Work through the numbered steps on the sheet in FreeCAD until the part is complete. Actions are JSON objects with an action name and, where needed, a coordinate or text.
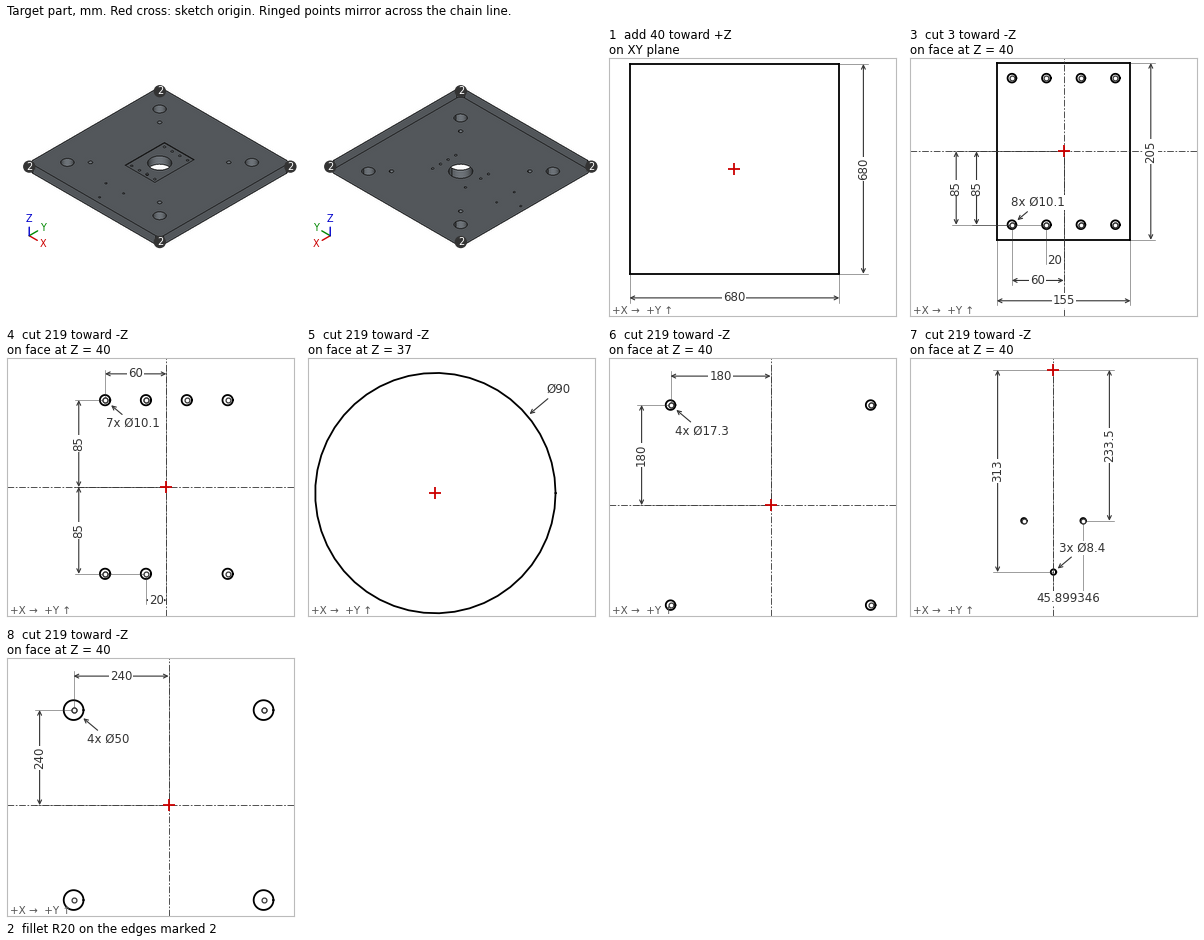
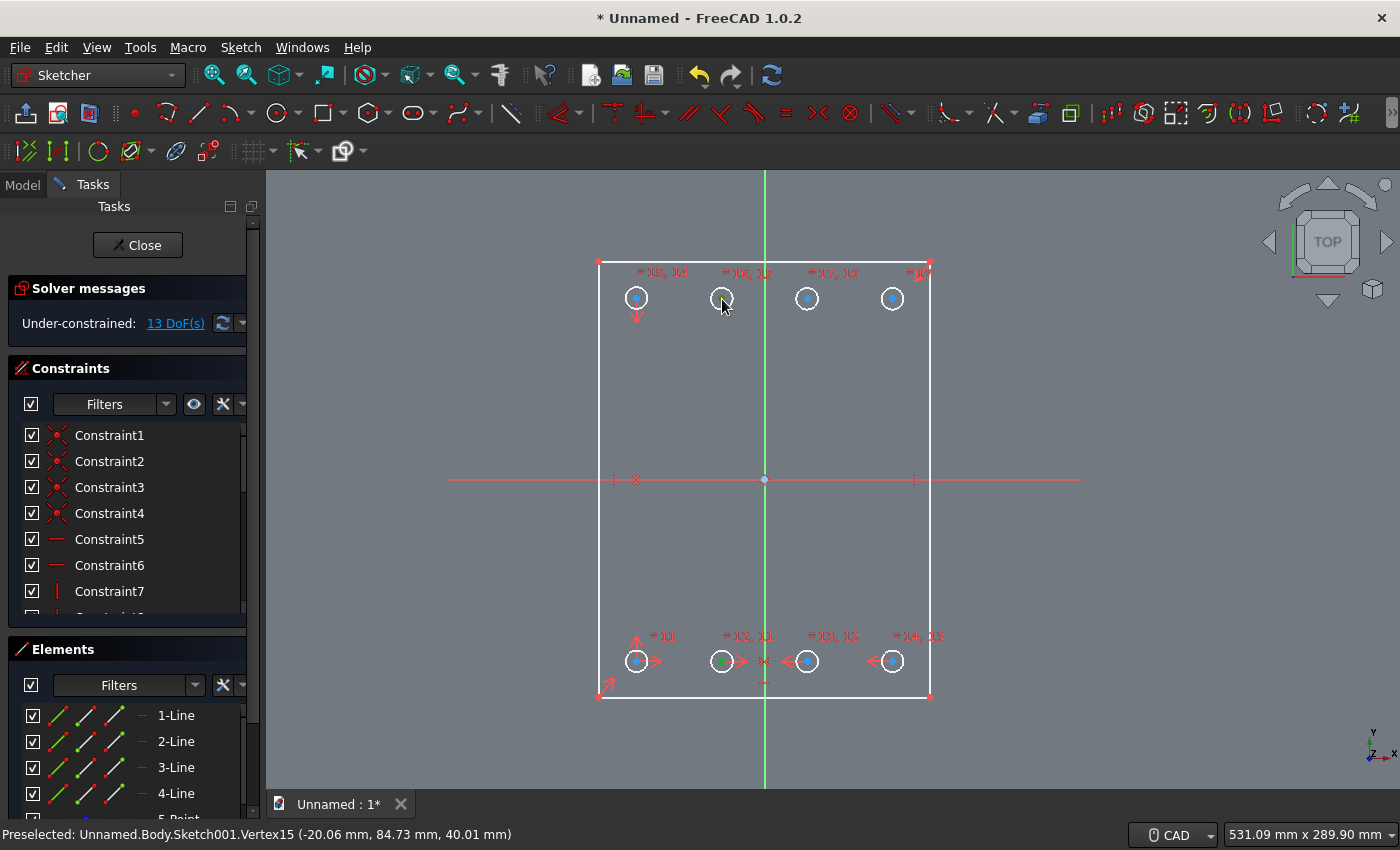
{"action": "left_click", "coordinate": [496, 480]}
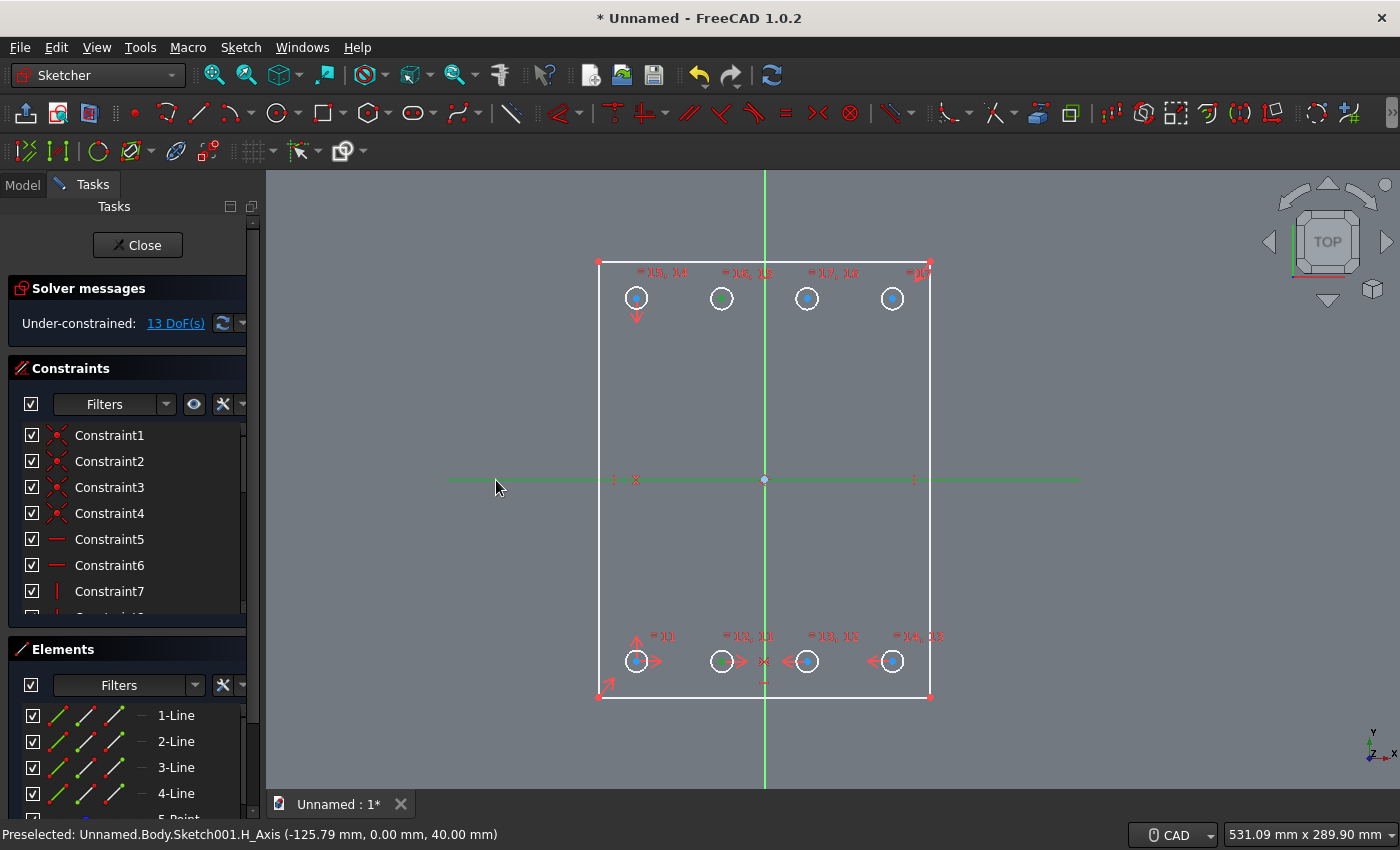
{"action": "left_click", "coordinate": [818, 114]}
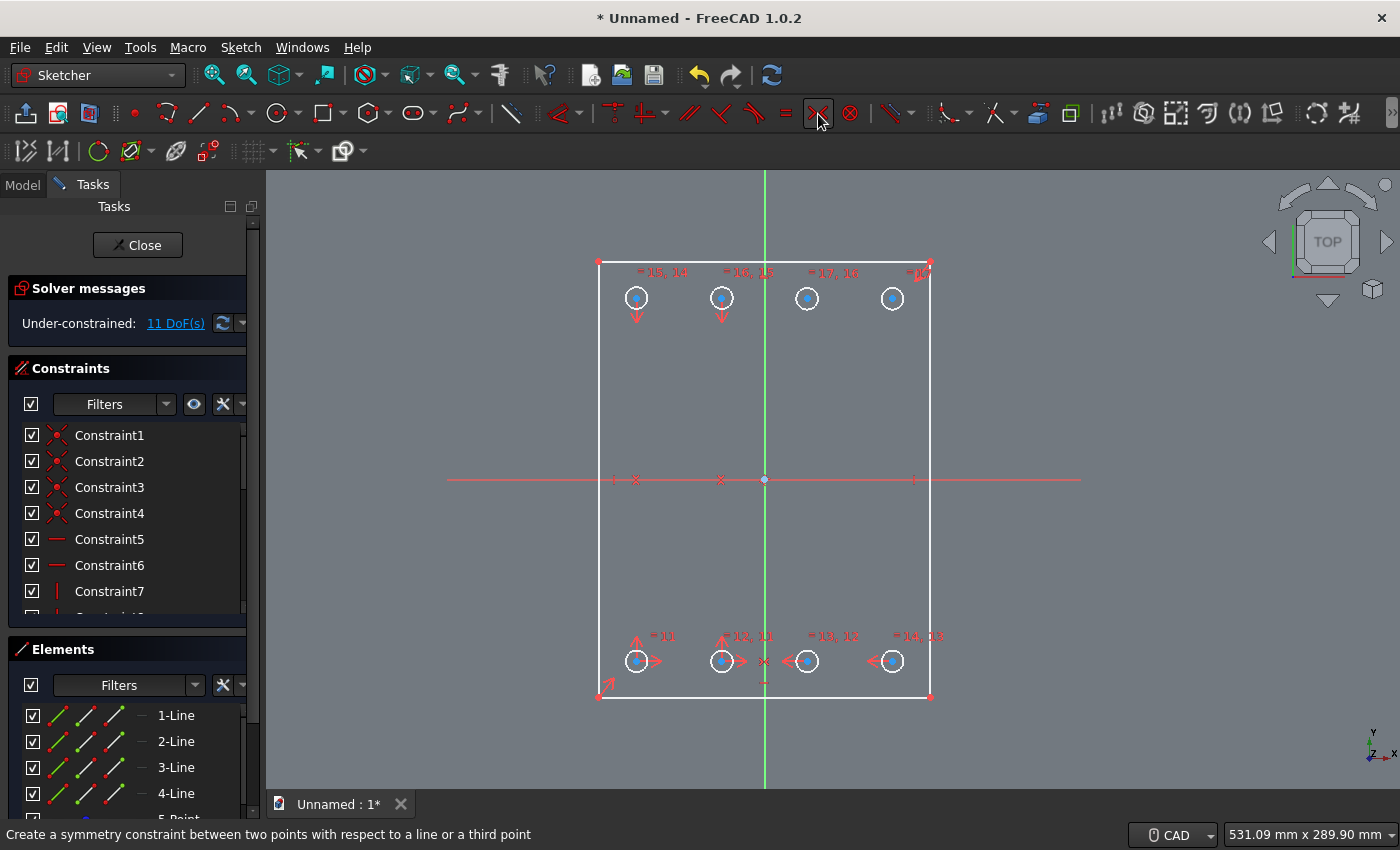
{"action": "left_click", "coordinate": [807, 661]}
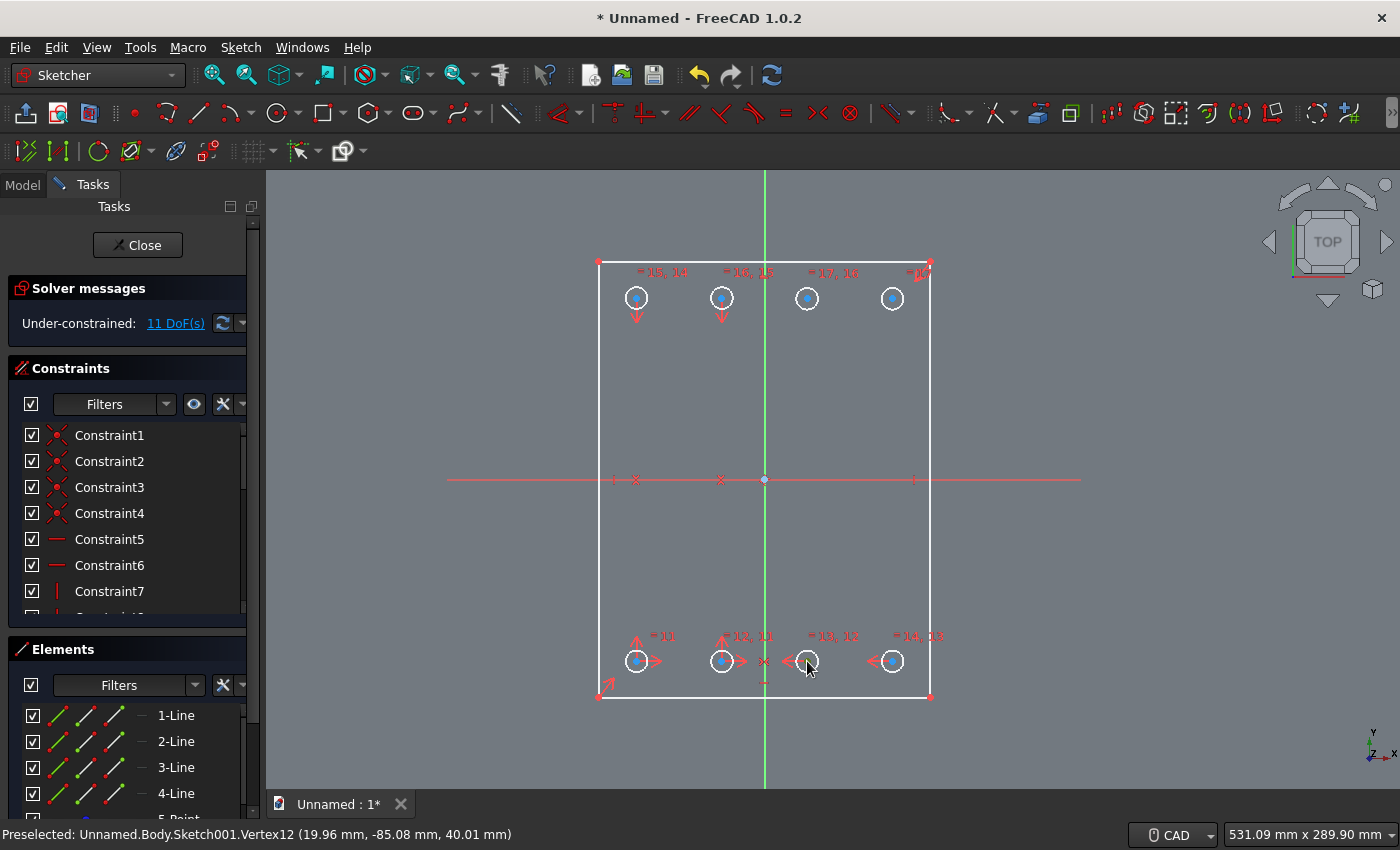
{"action": "left_click", "coordinate": [807, 299]}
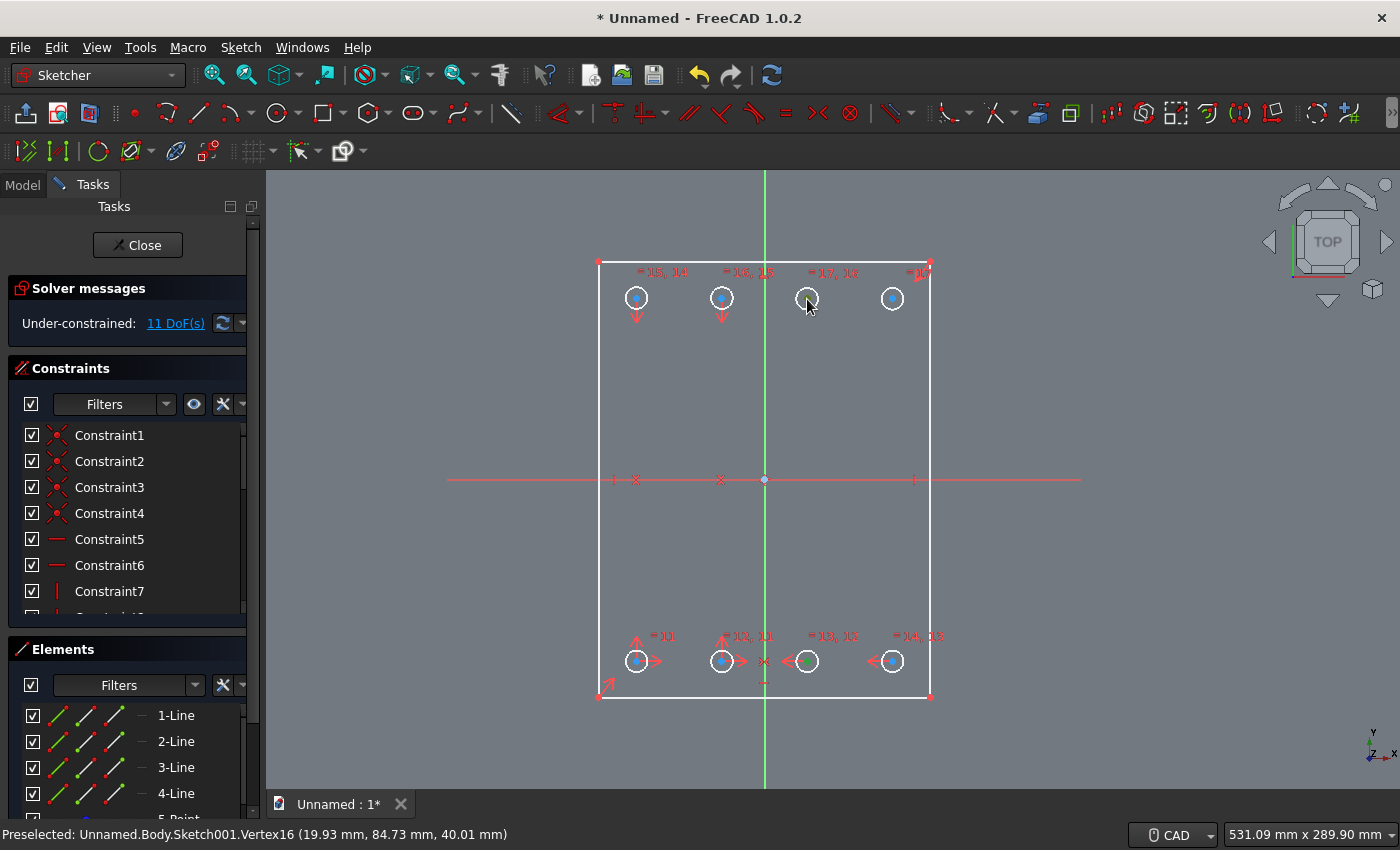
{"action": "left_click", "coordinate": [496, 480]}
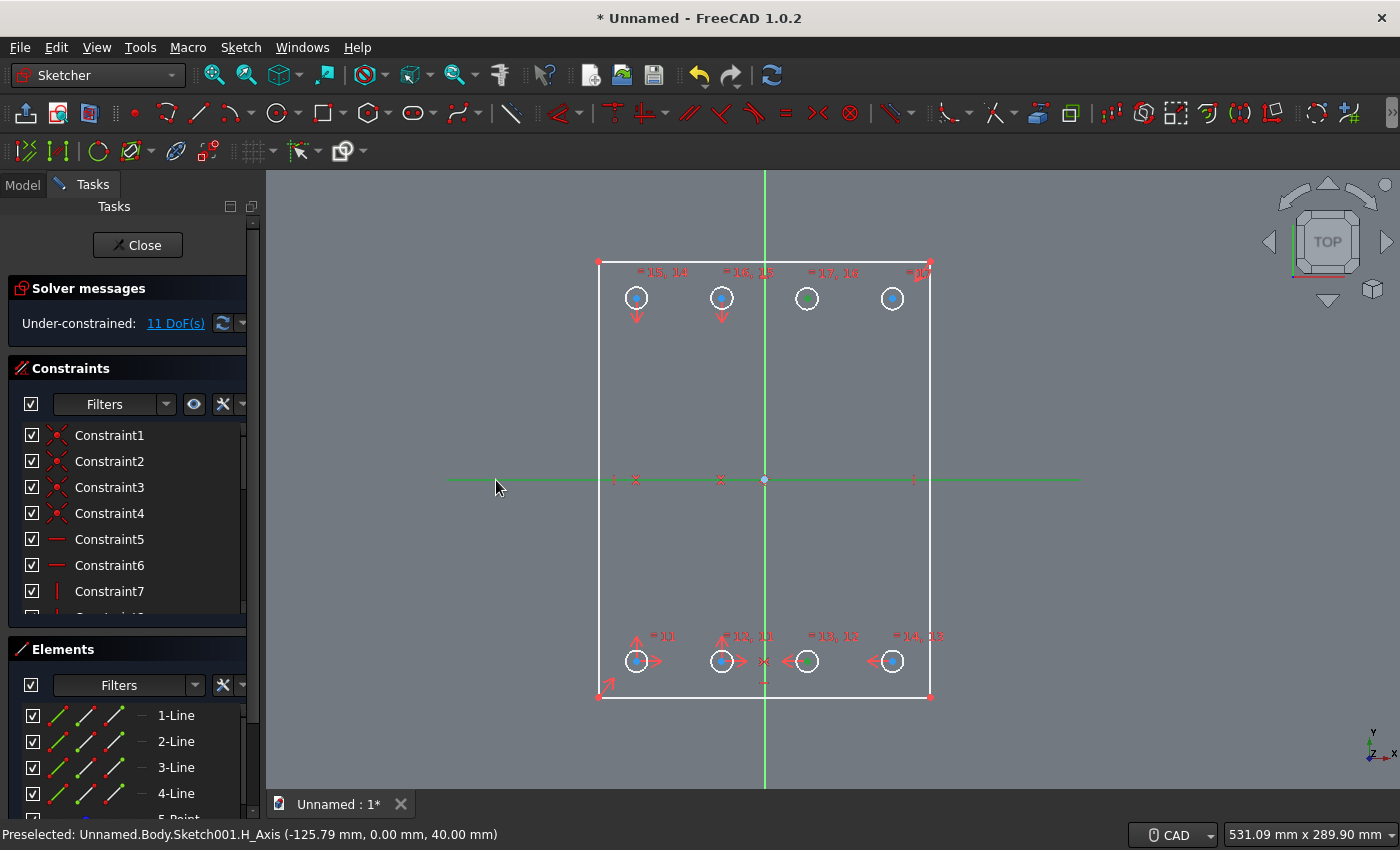
{"action": "left_click", "coordinate": [818, 114]}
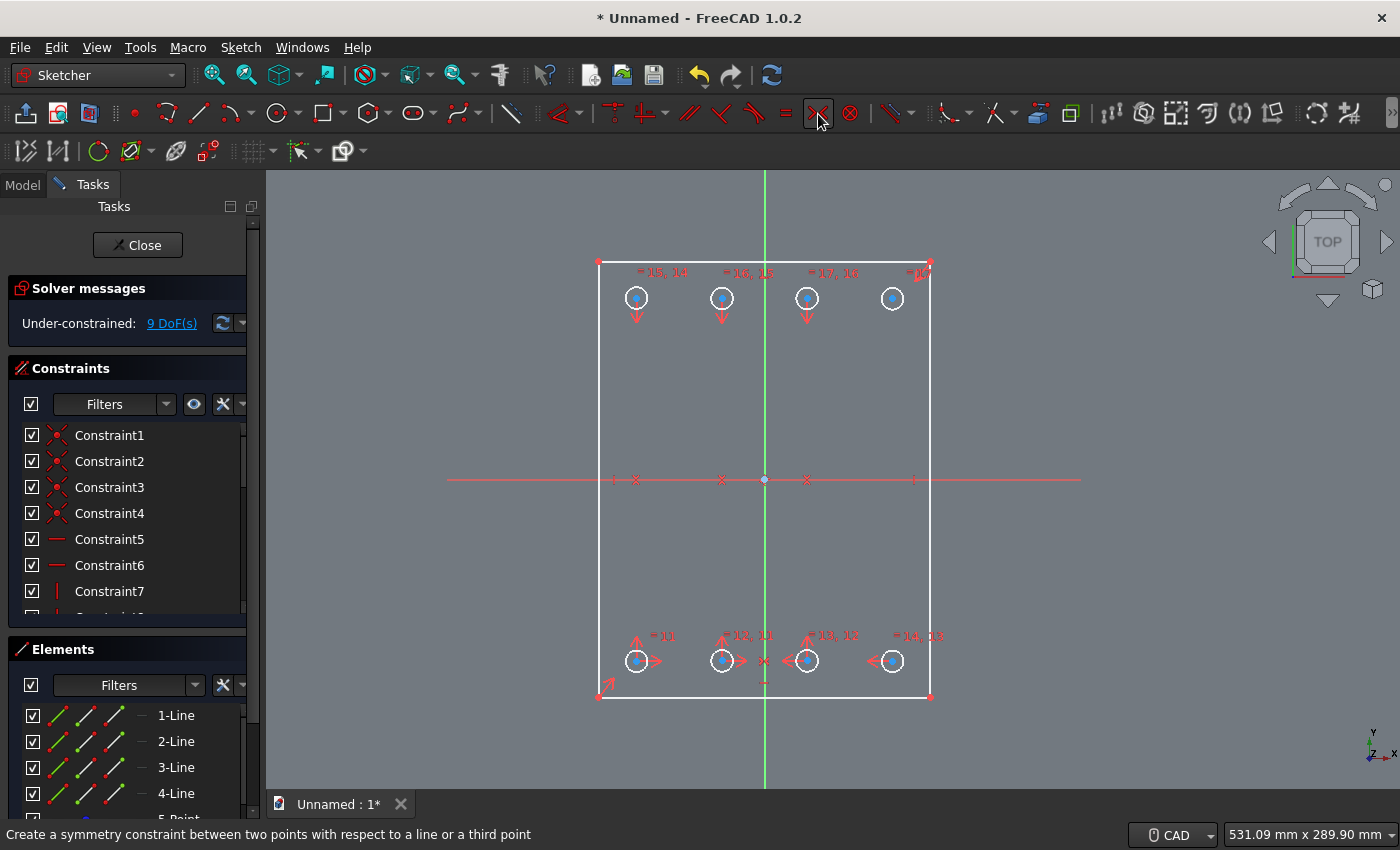
{"action": "left_click", "coordinate": [893, 661]}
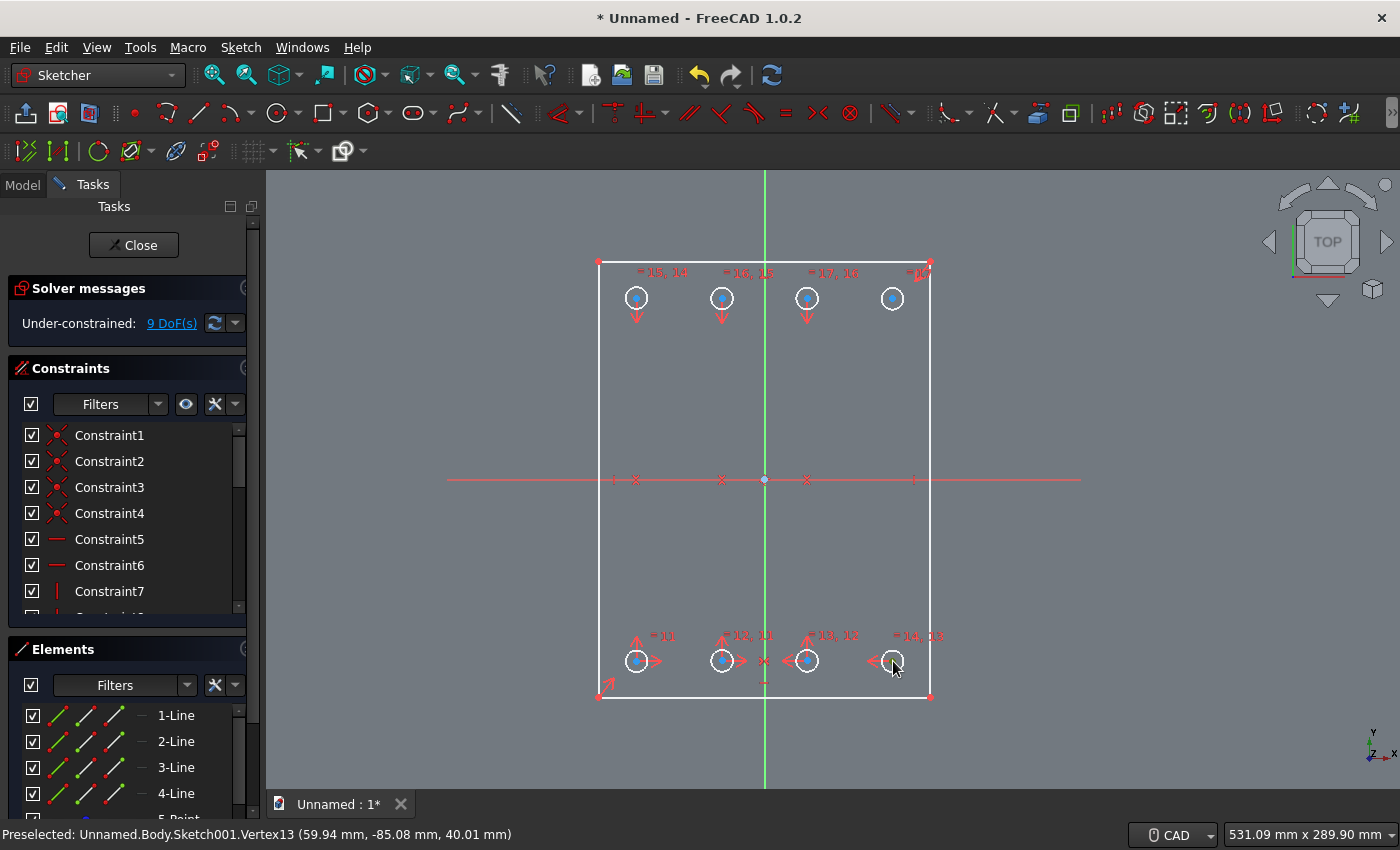
{"action": "left_click", "coordinate": [893, 299]}